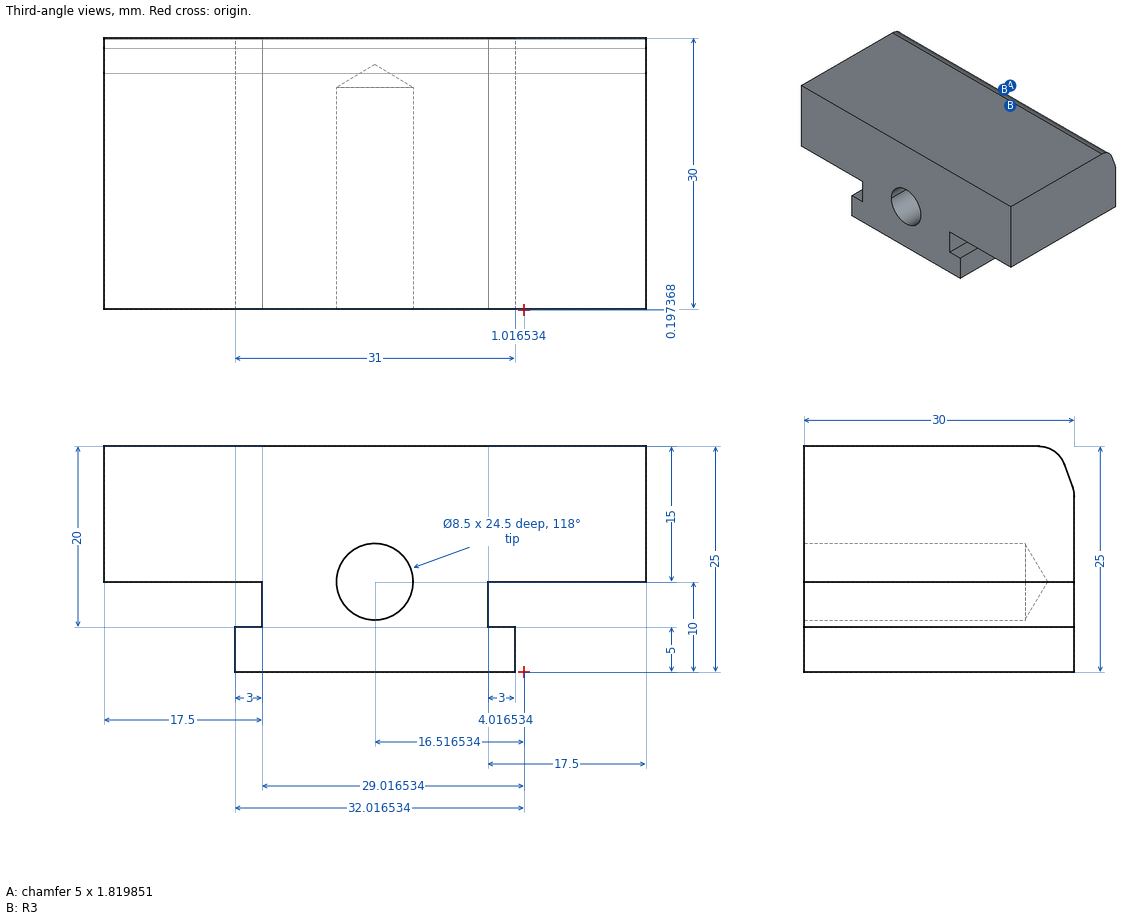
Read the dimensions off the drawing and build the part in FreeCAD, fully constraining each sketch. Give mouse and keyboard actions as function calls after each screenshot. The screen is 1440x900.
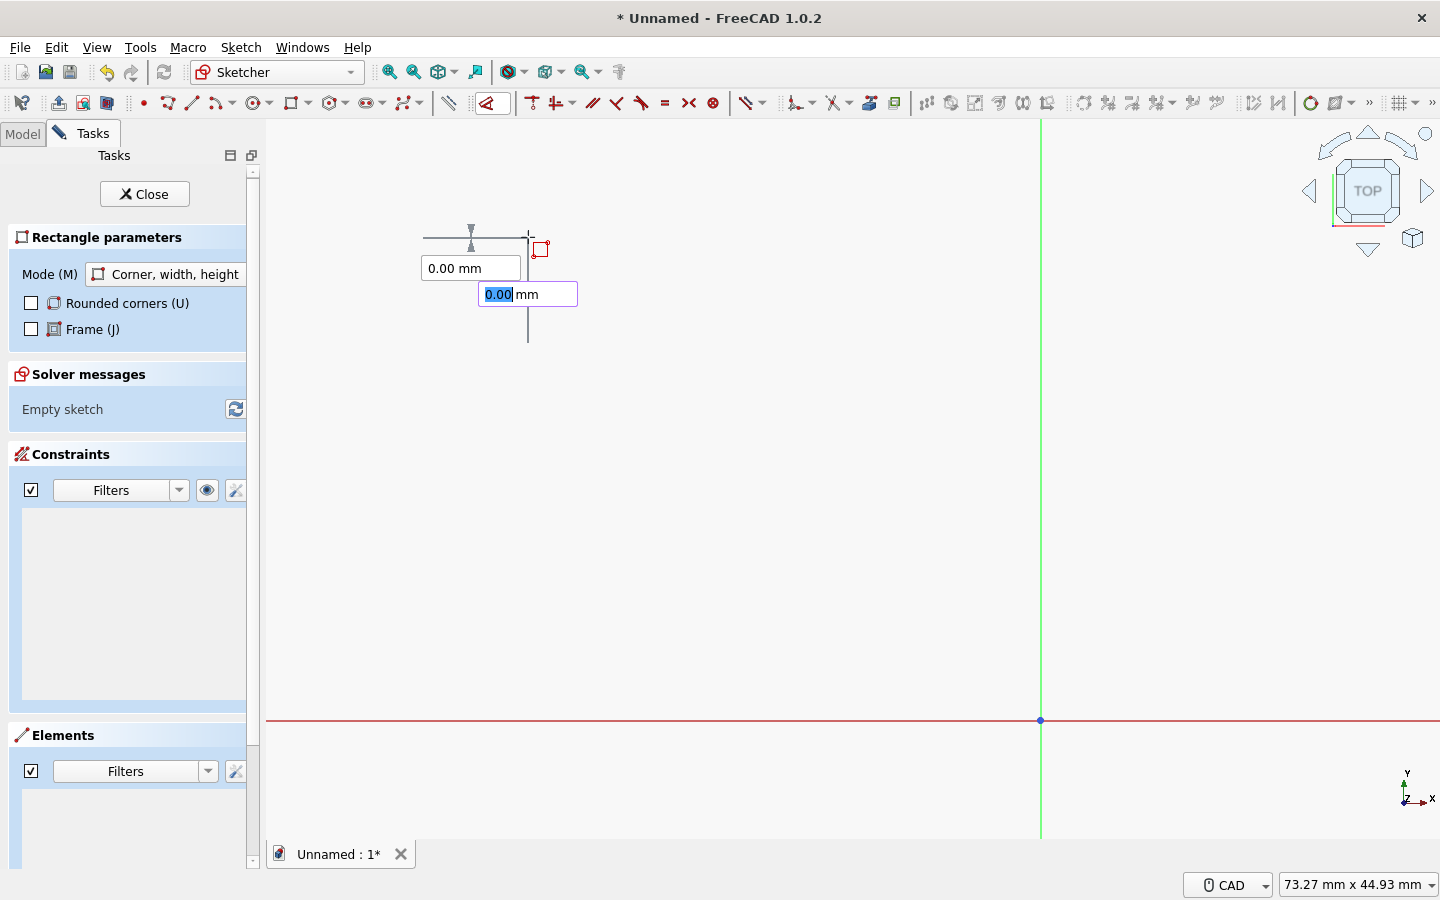
scroll(1024, 718, up, 9)
move(1024, 711)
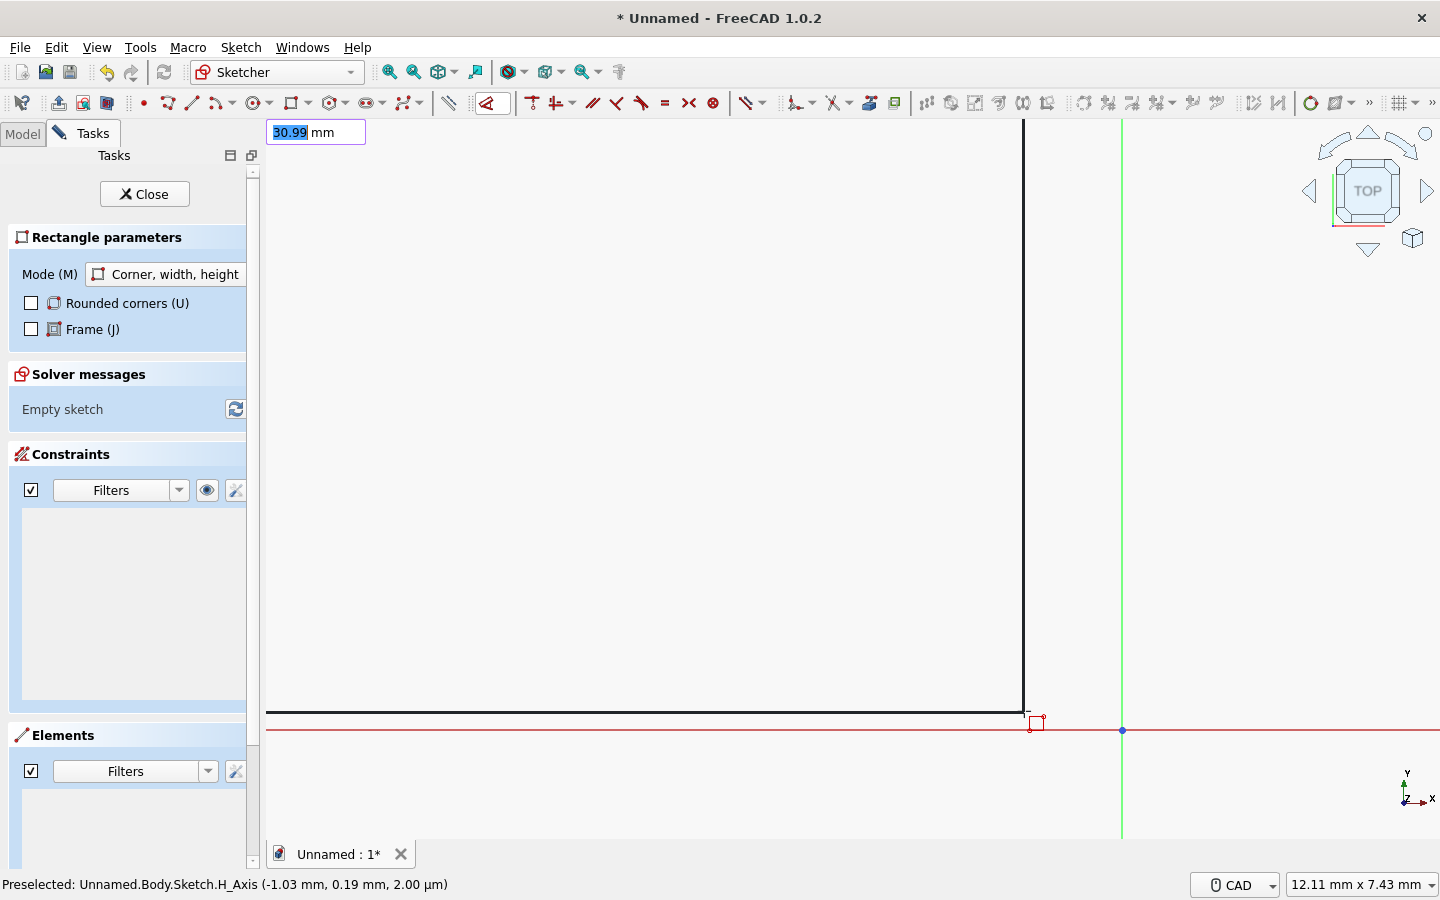
text(31)
key(Tab)
text(30)
key(Return)
key(Escape)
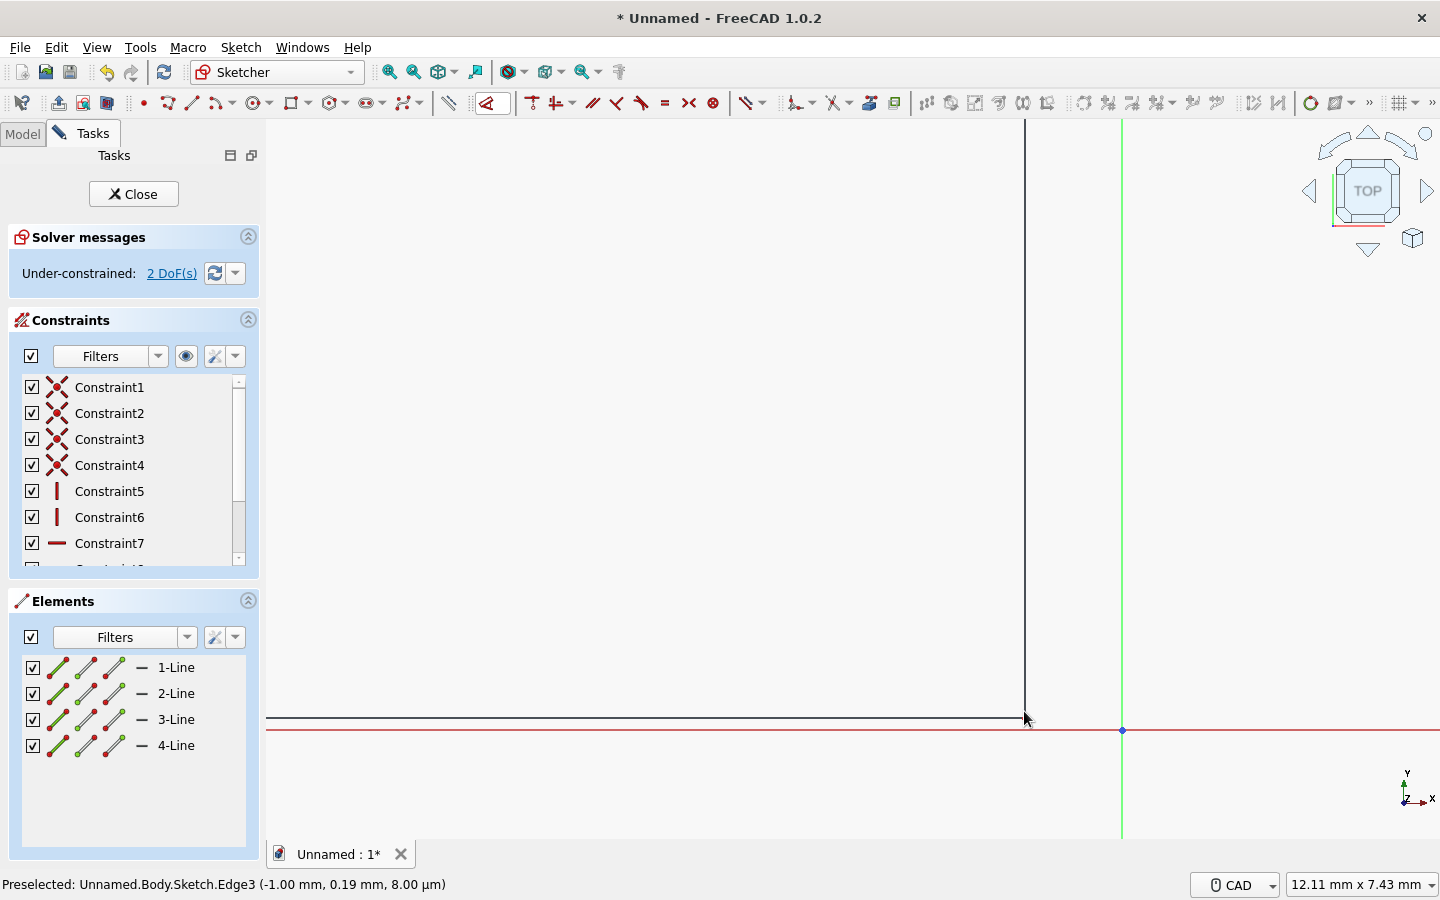
click(486, 104)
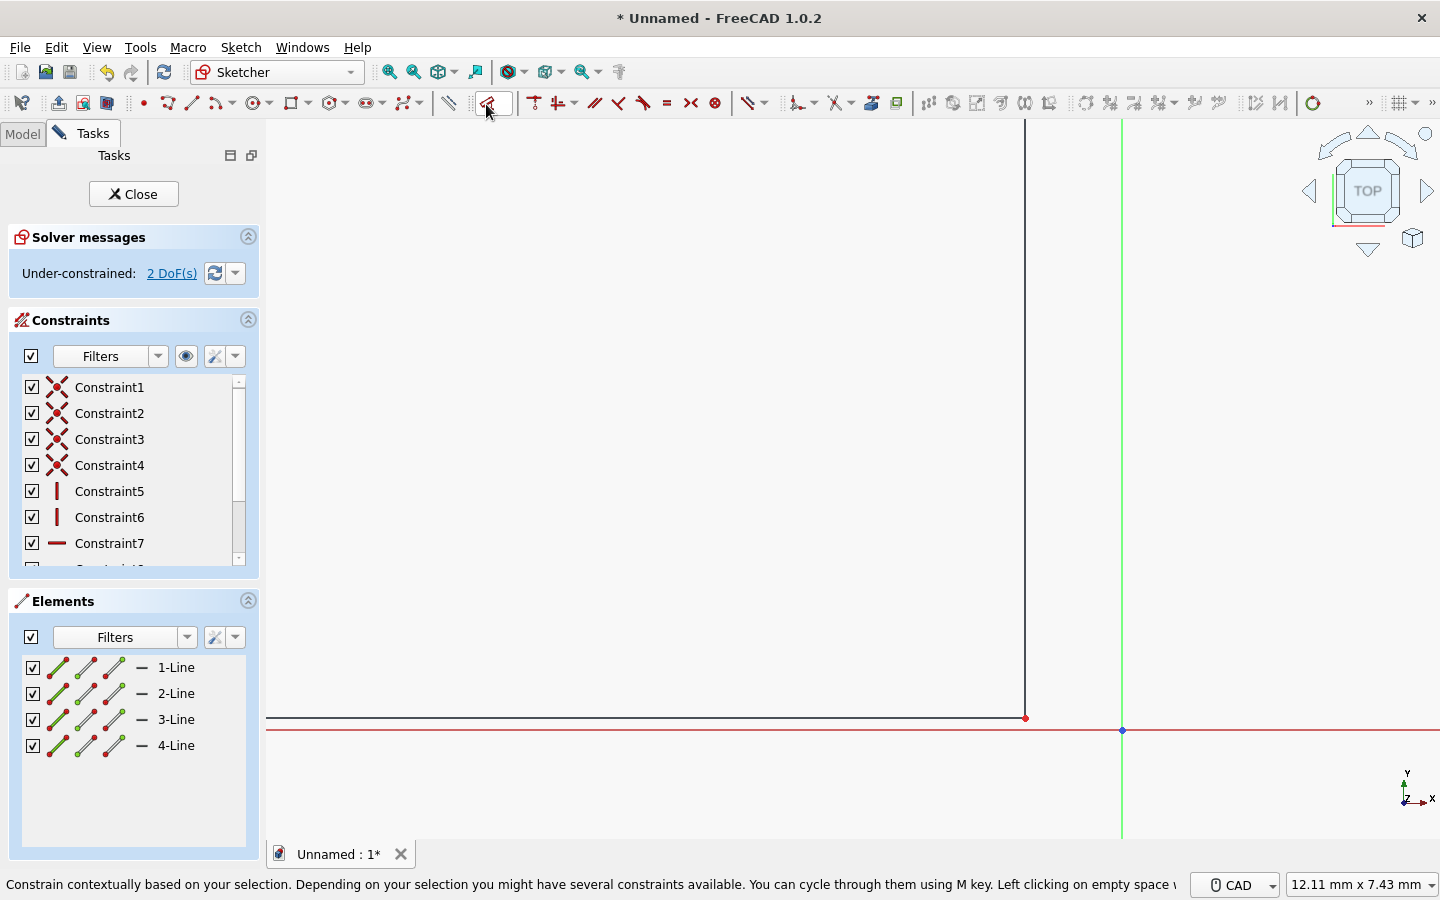
scroll(1025, 719, down, 9)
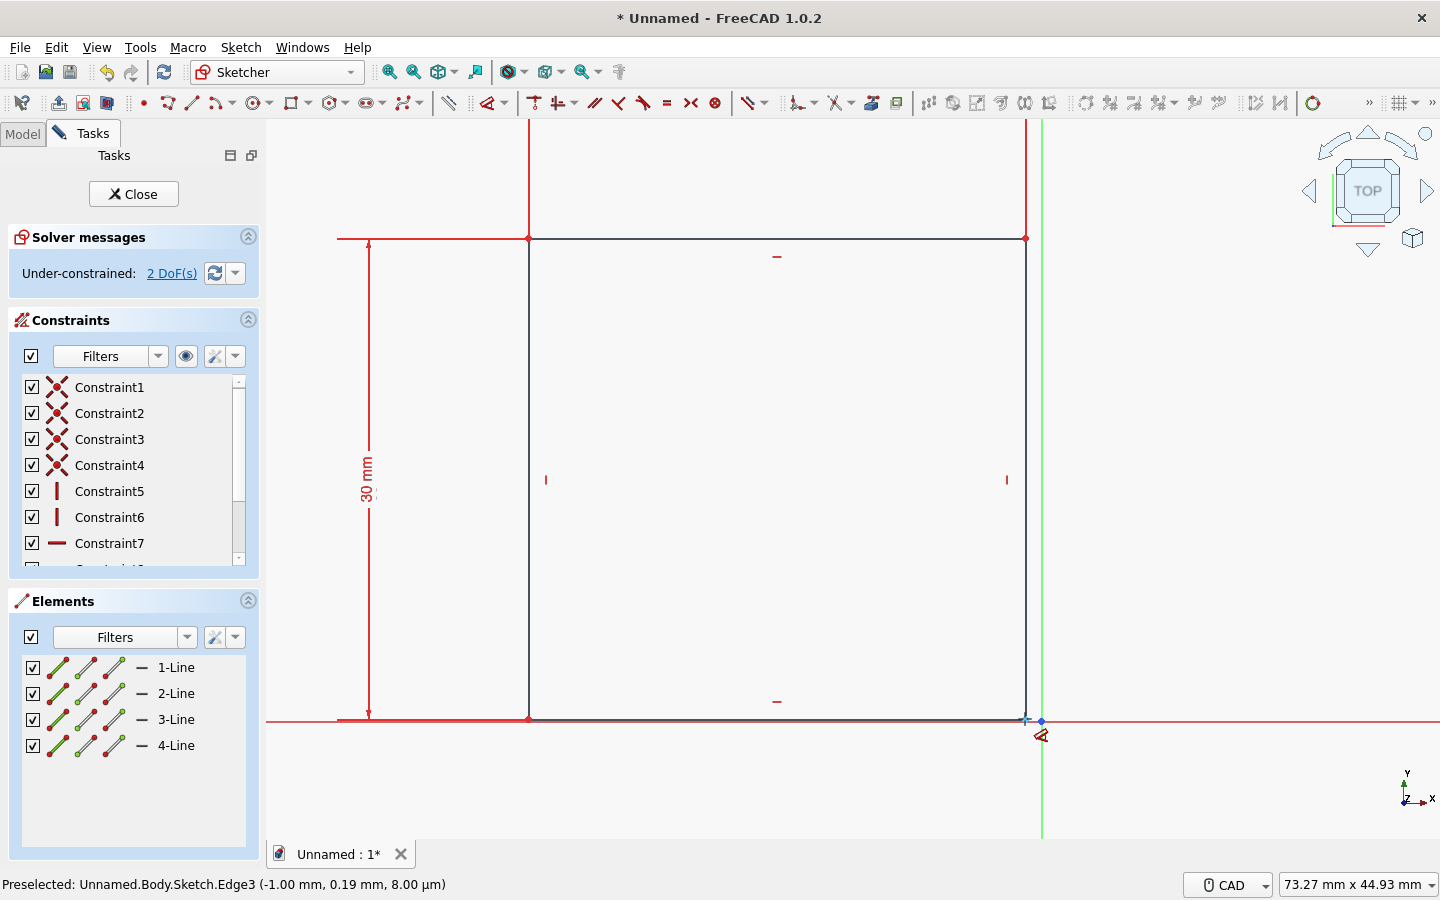
scroll(529, 720, up, 13)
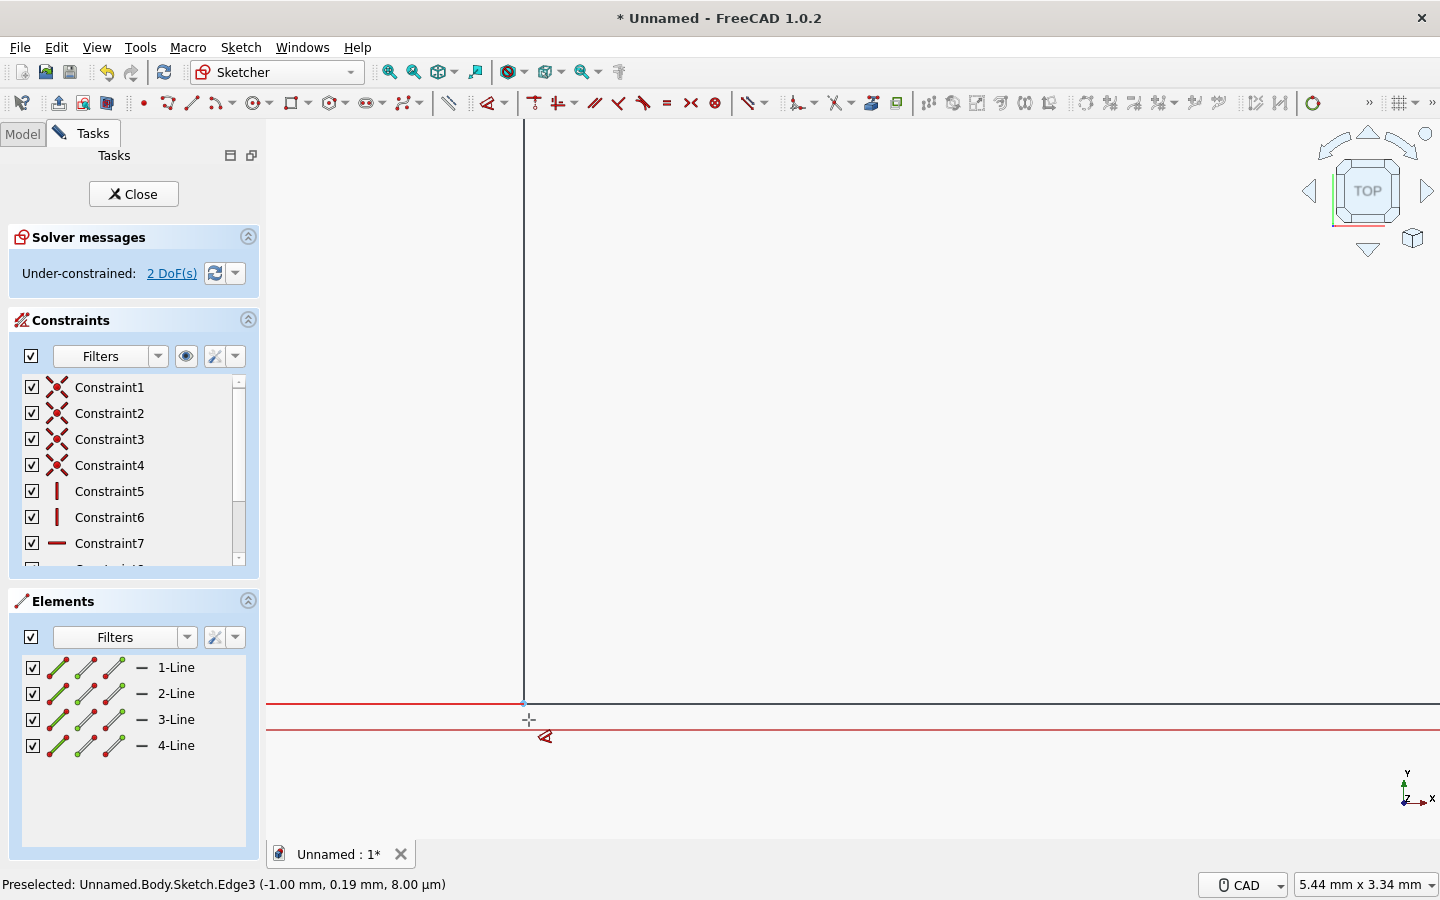
click(524, 704)
click(490, 717)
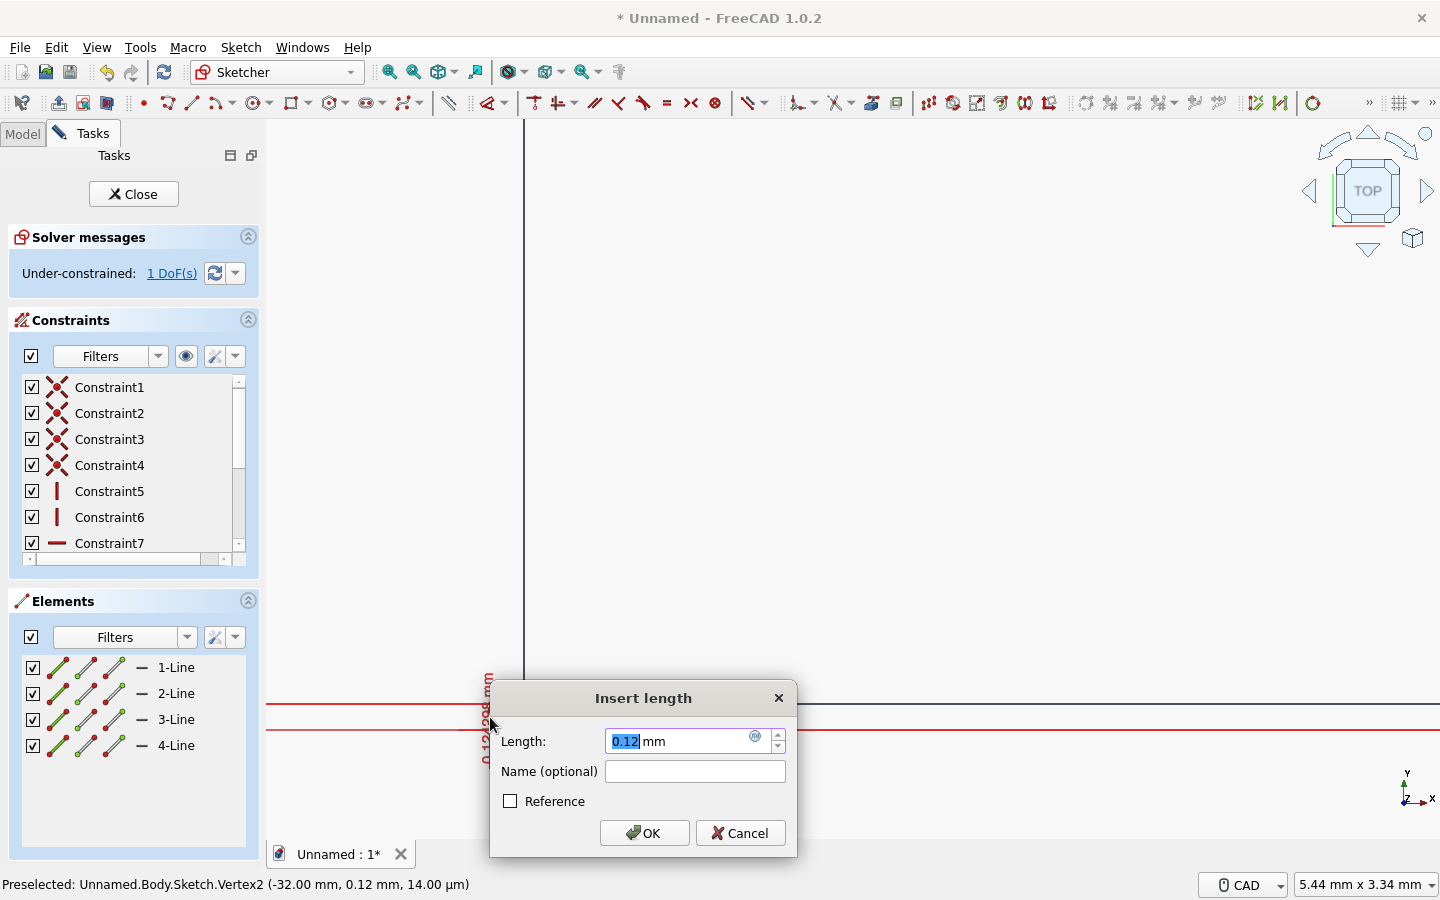
text(0.197368)
key(Return)